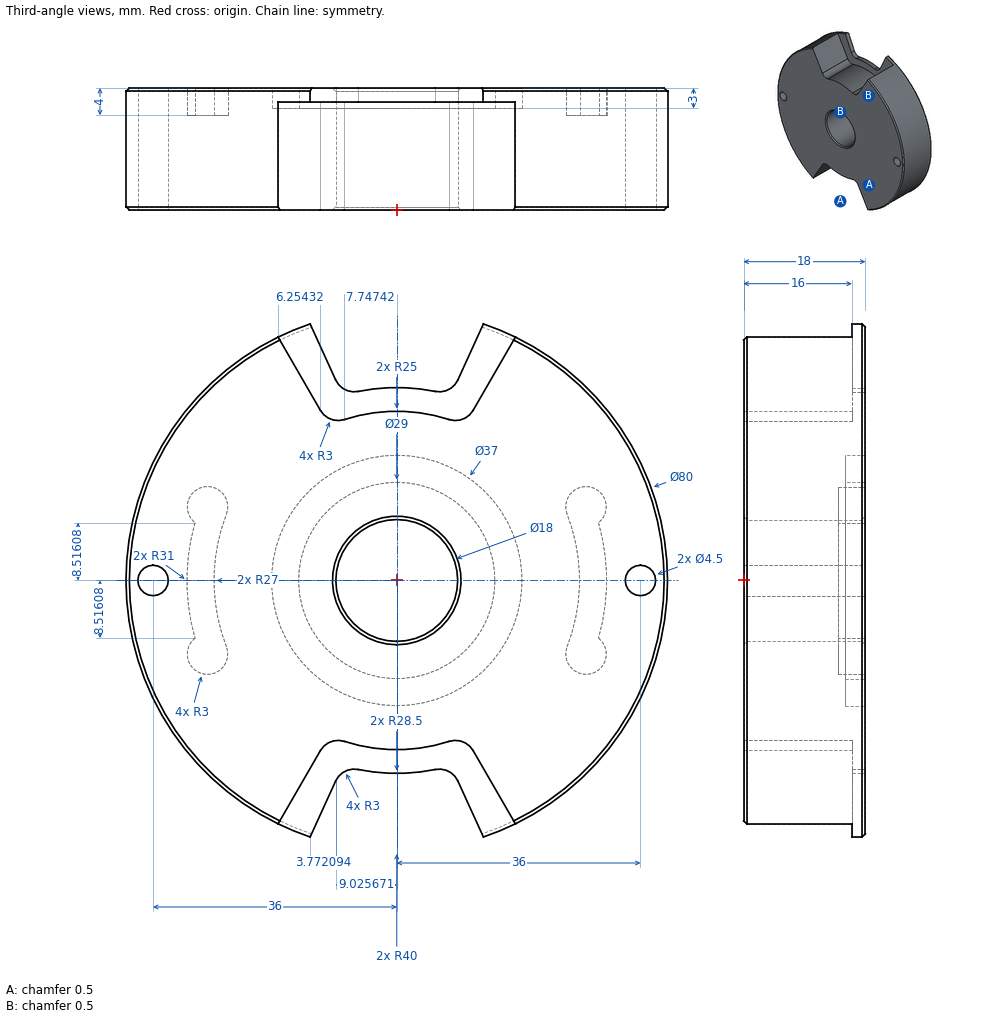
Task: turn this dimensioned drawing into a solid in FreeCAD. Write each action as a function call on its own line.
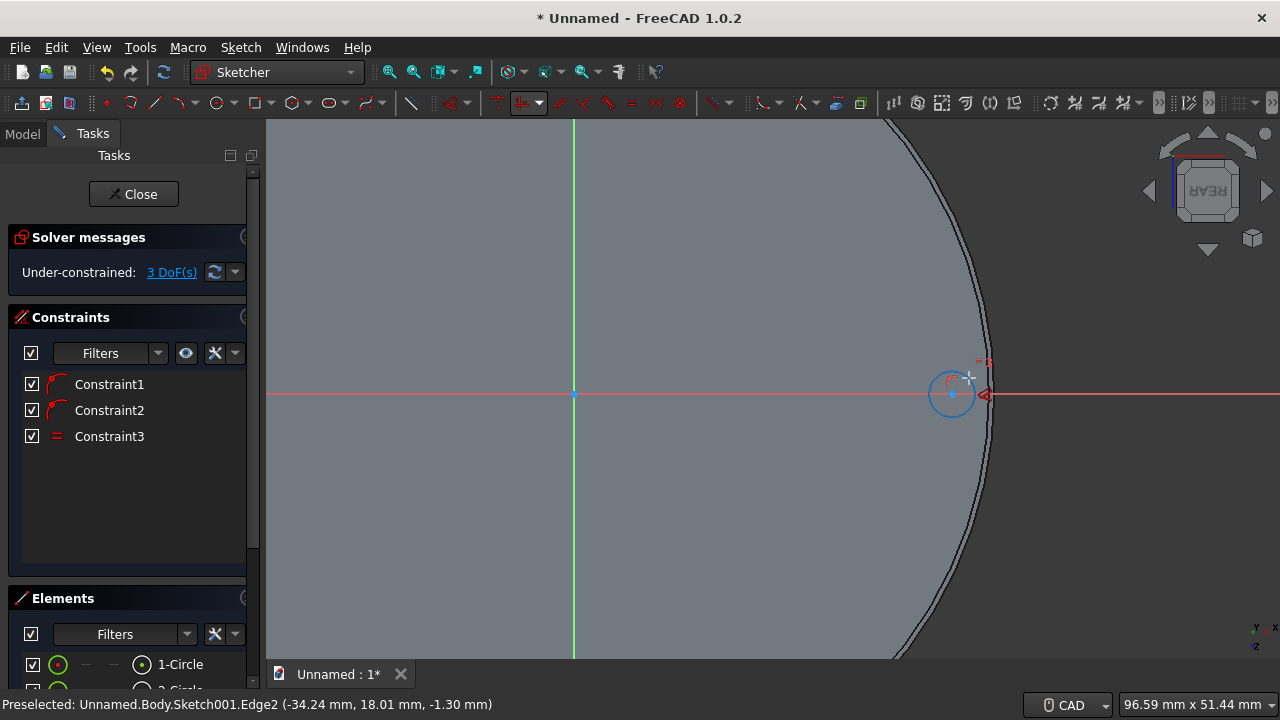
click(968, 378)
click(990, 355)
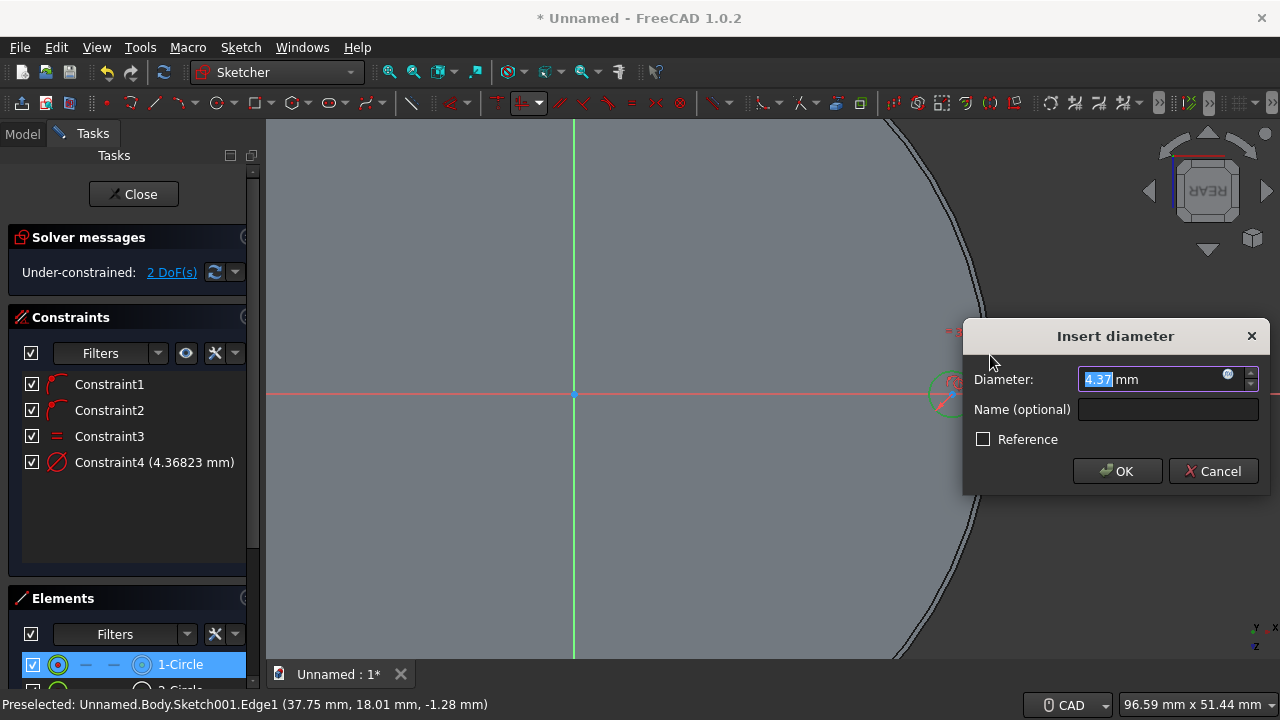
text(4.5)
key(Return)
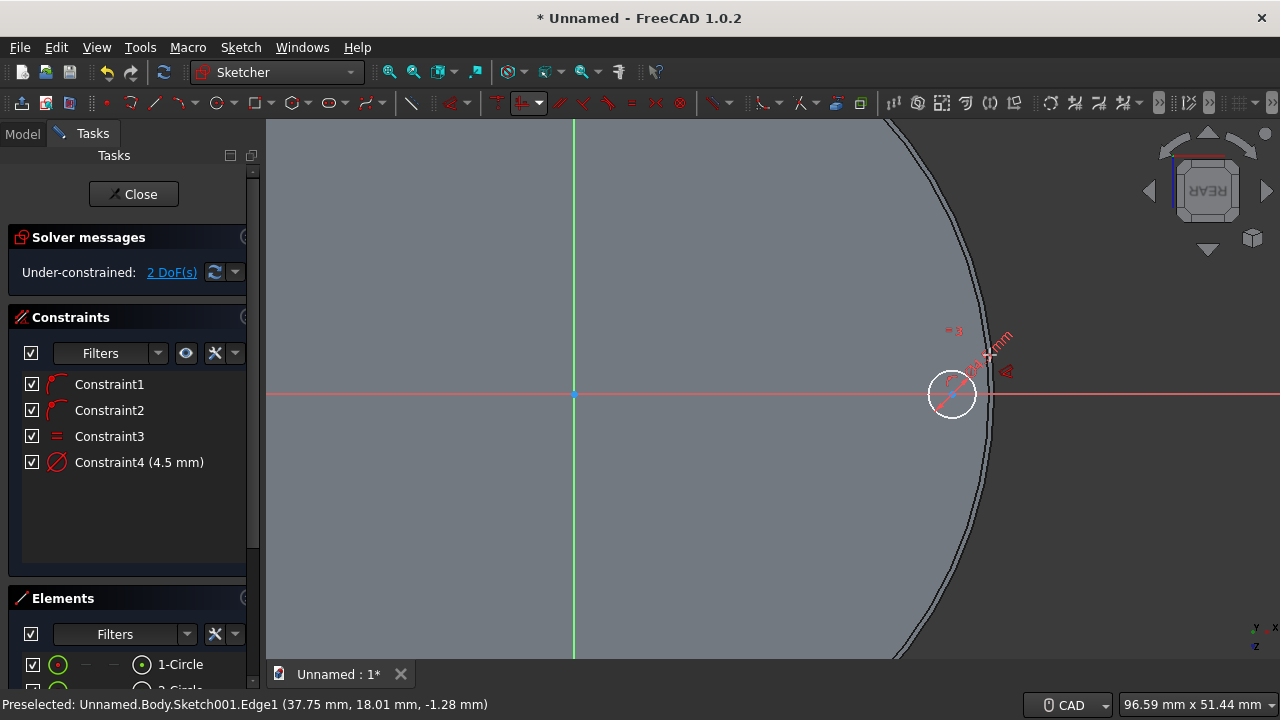
click(952, 394)
click(763, 428)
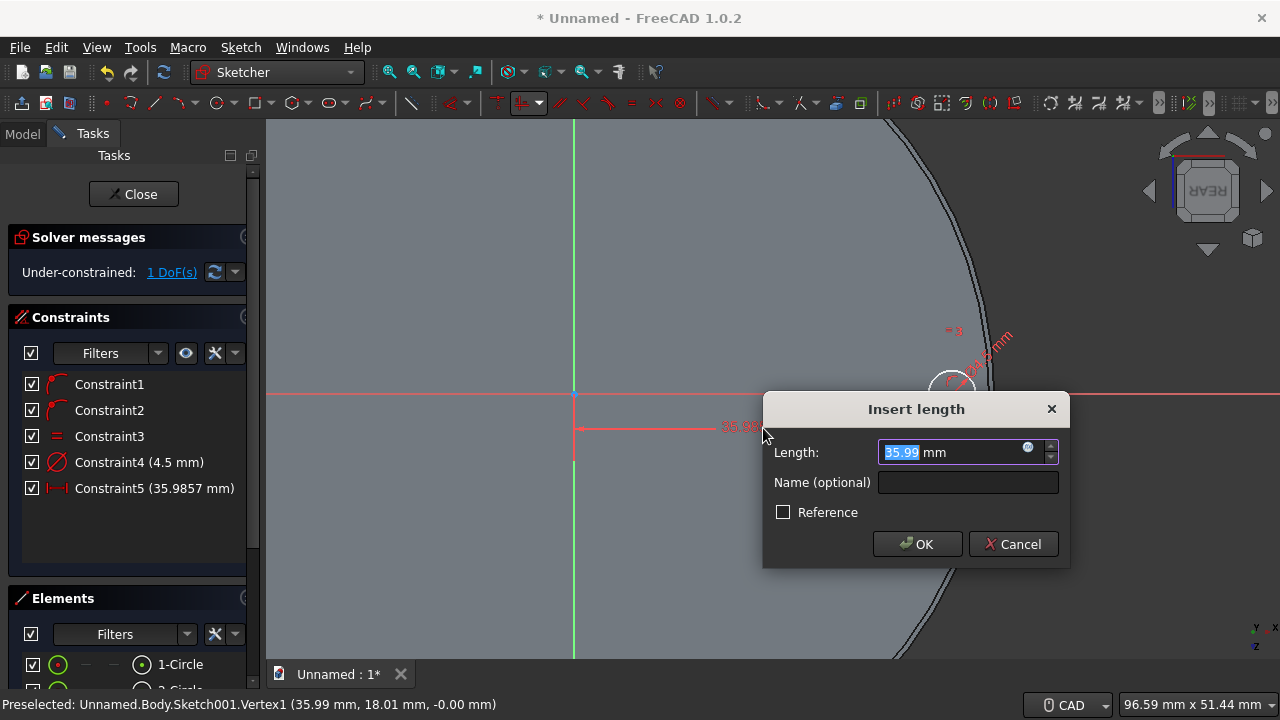
text(36)
key(Return)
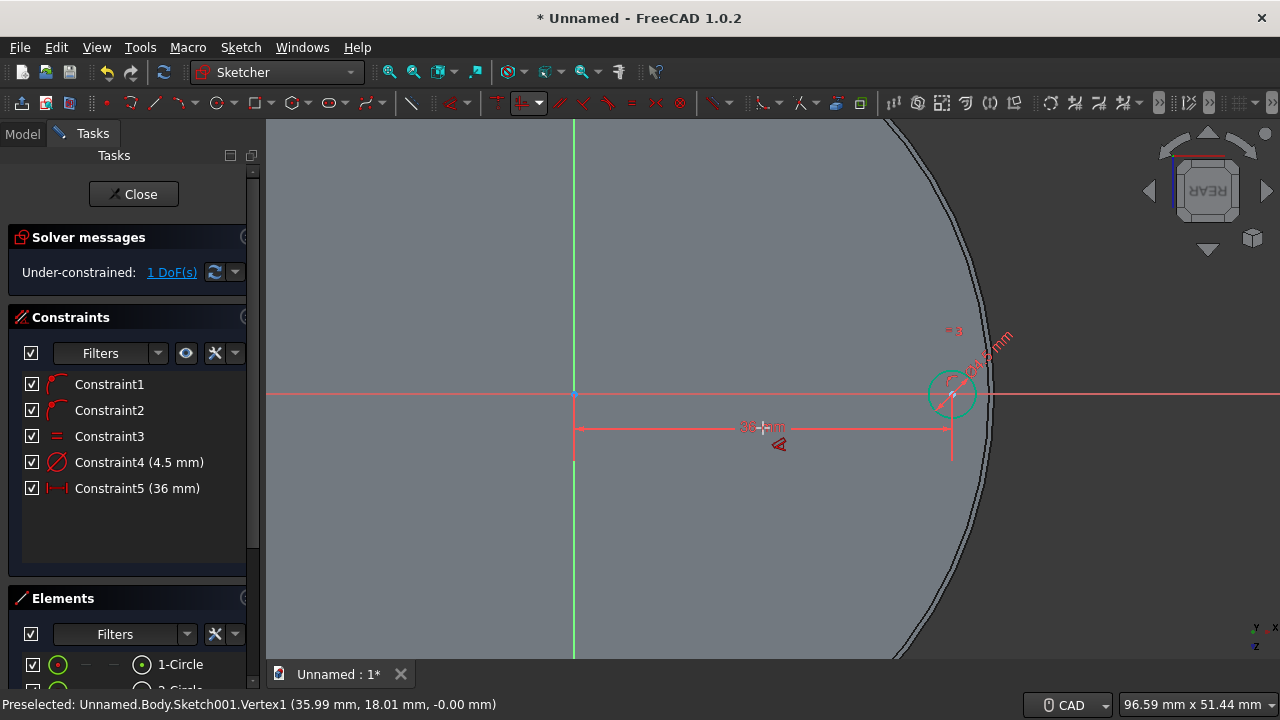
scroll(969, 378, down, 2)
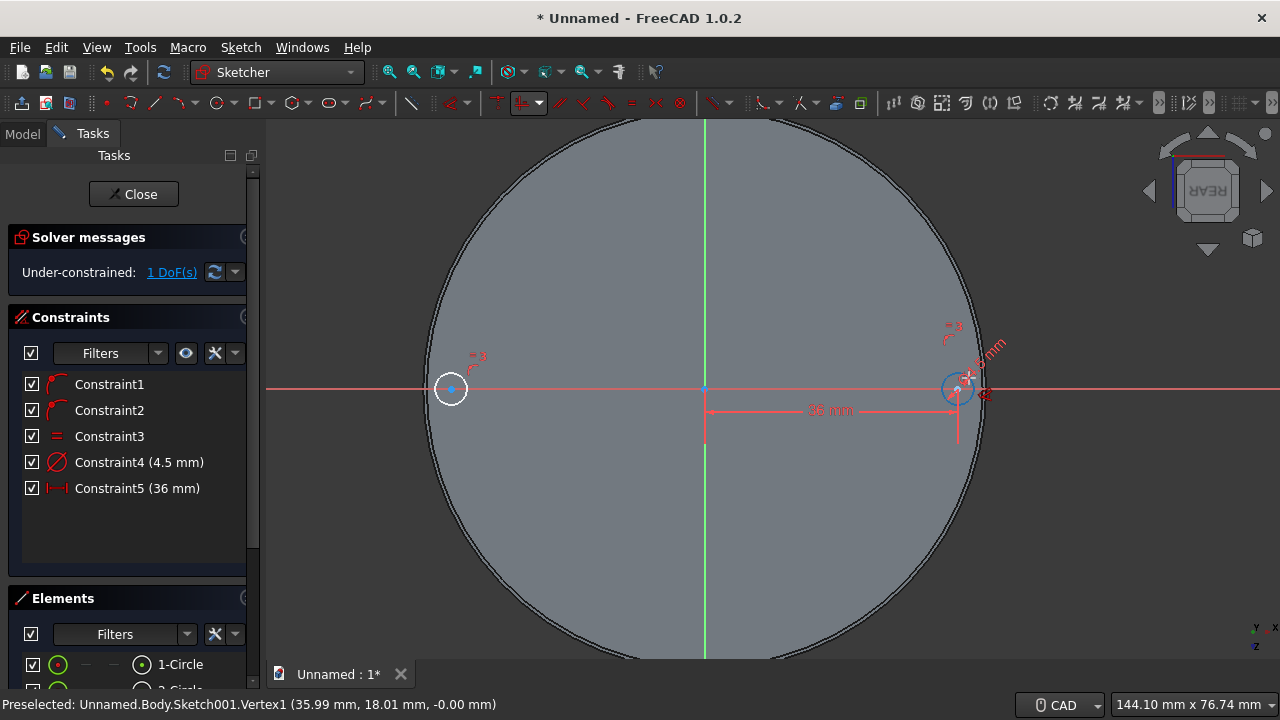
click(451, 389)
click(578, 423)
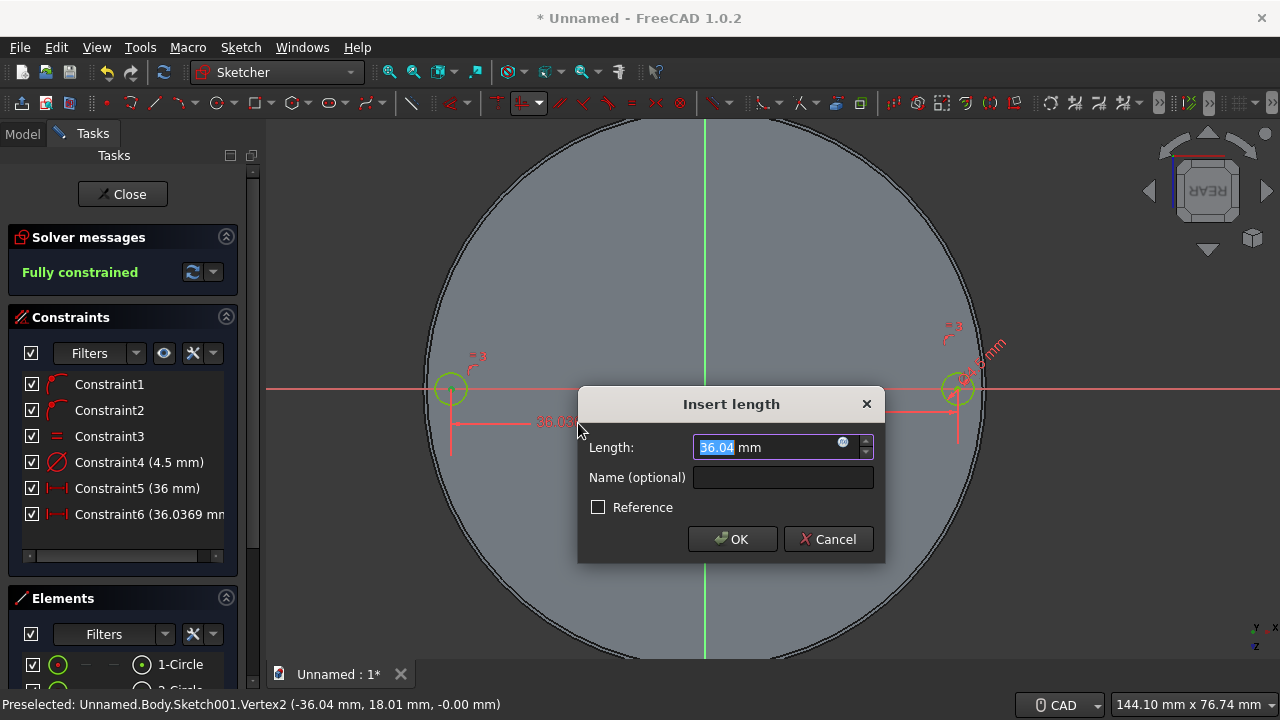
text(36)
key(Return)
key(Escape)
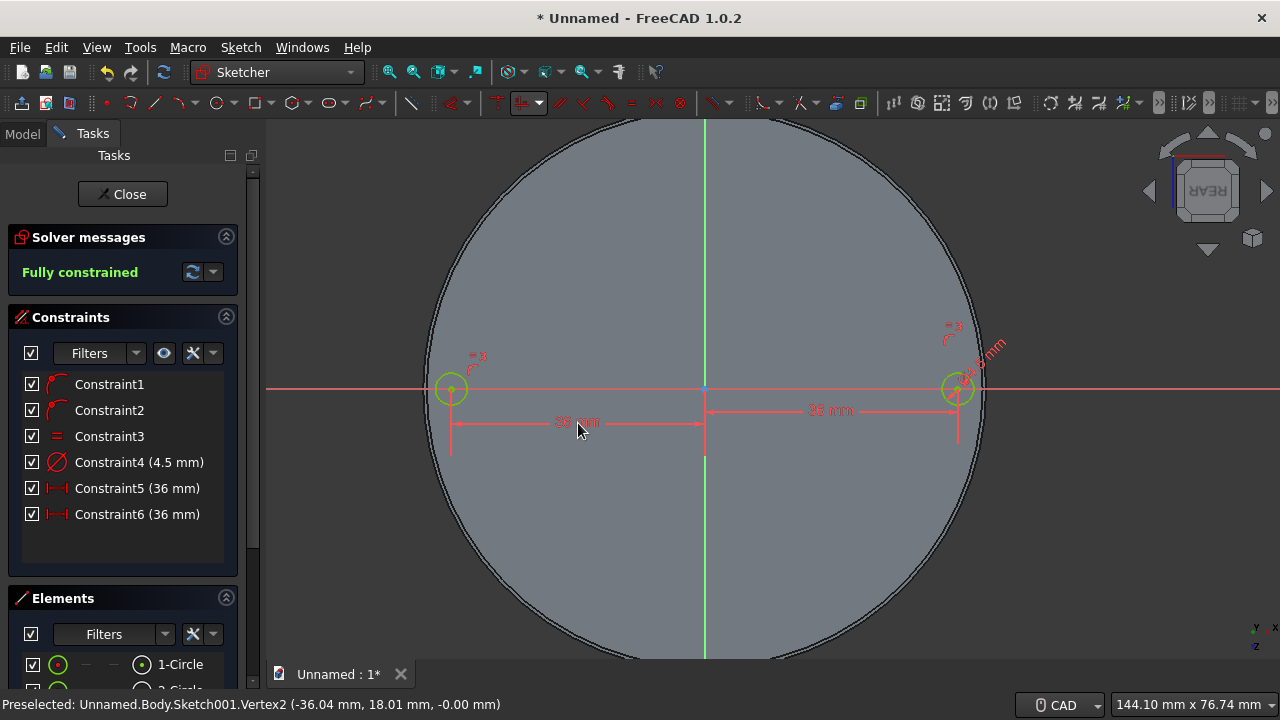
click(123, 194)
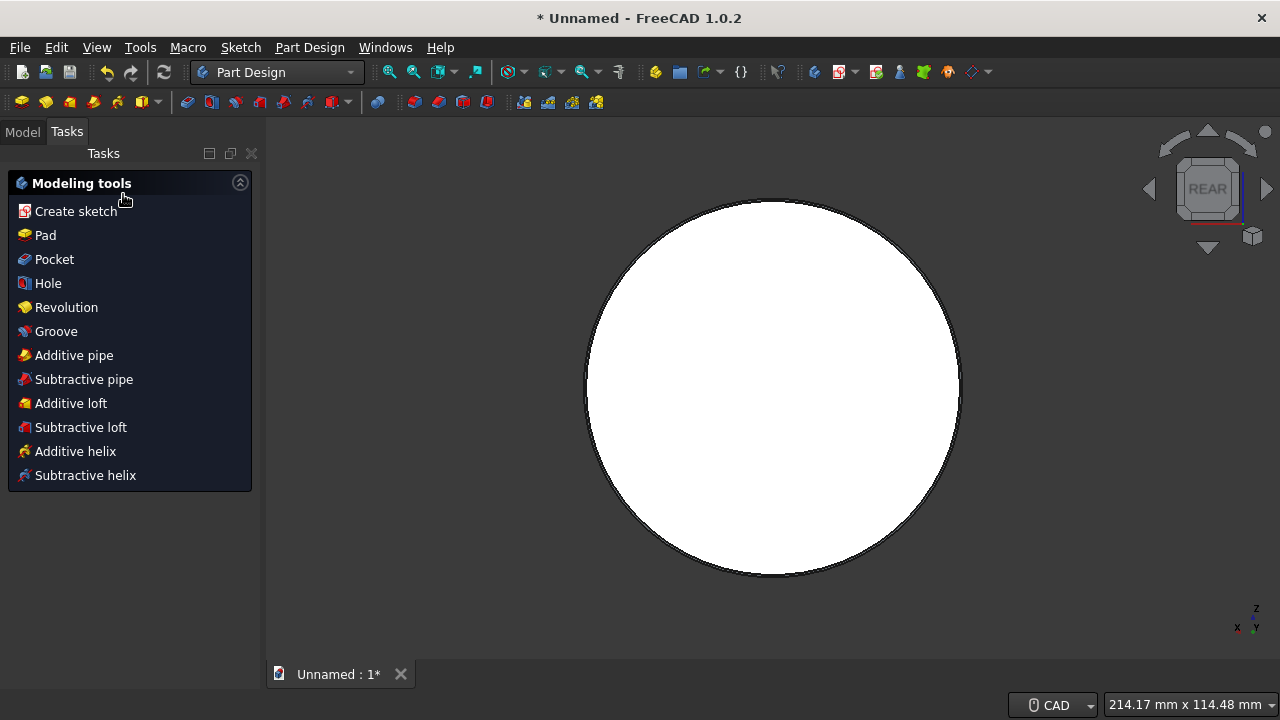
click(188, 102)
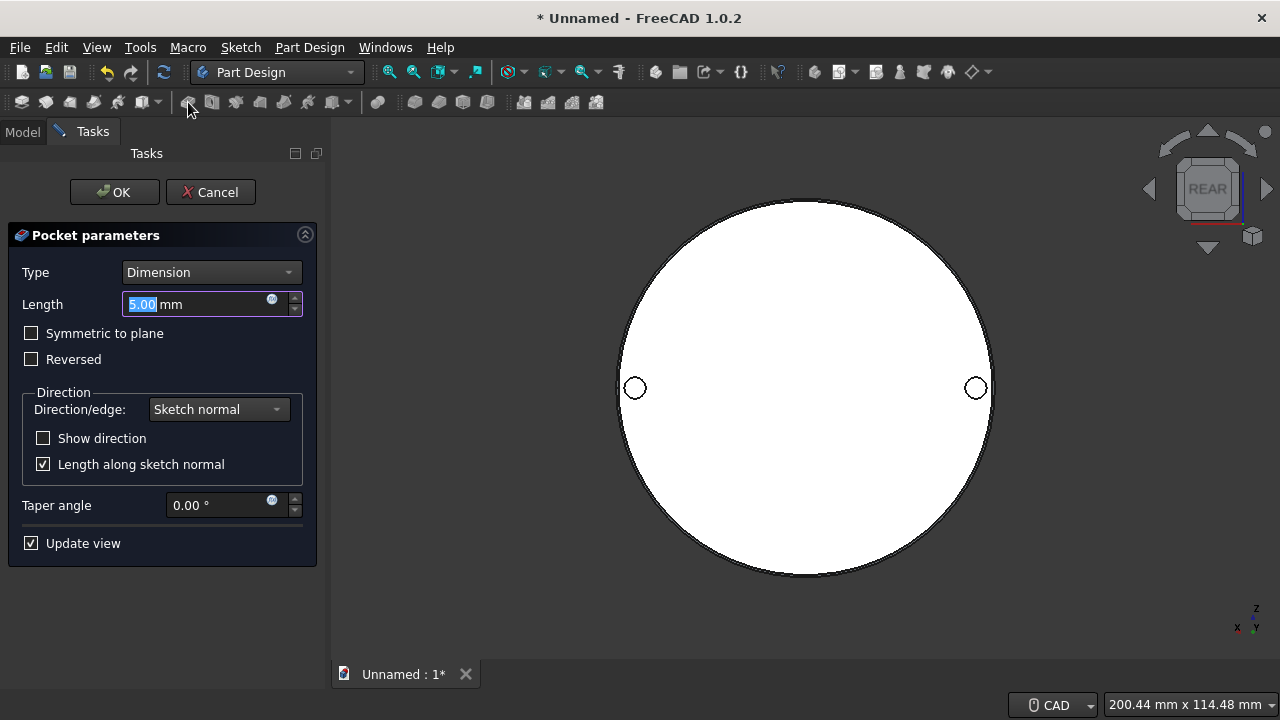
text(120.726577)
key(Tab)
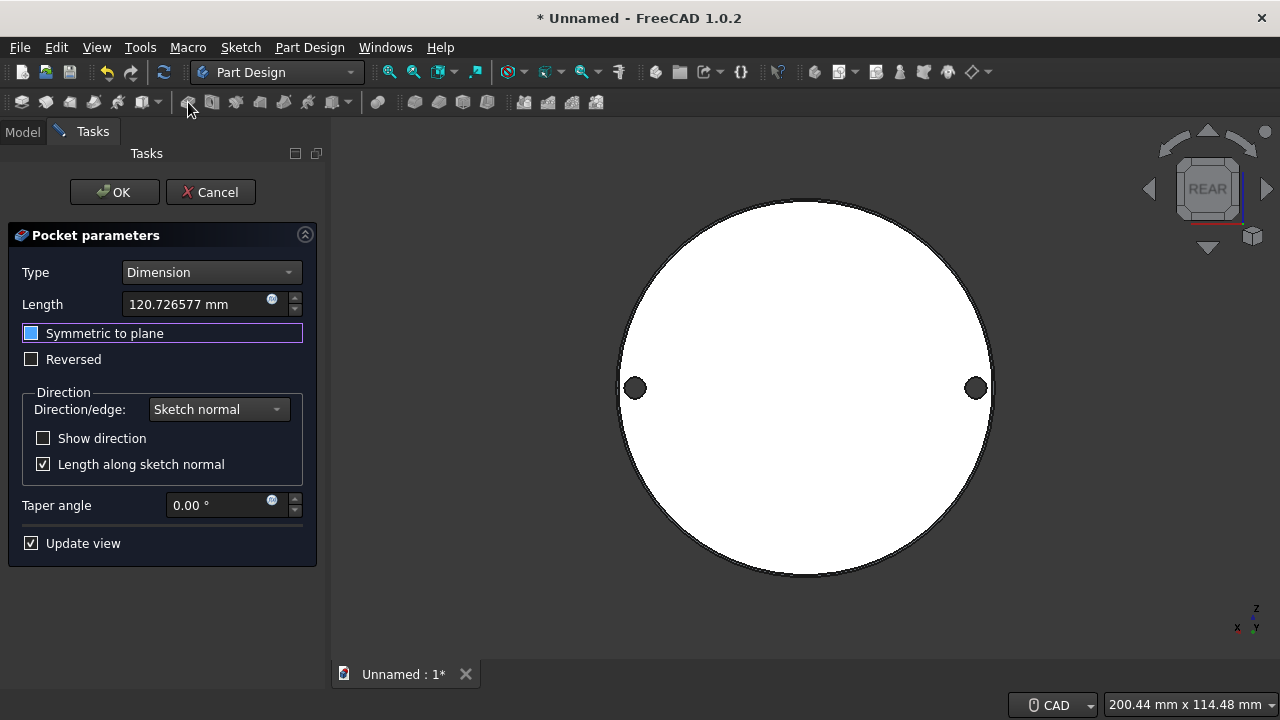
click(30, 333)